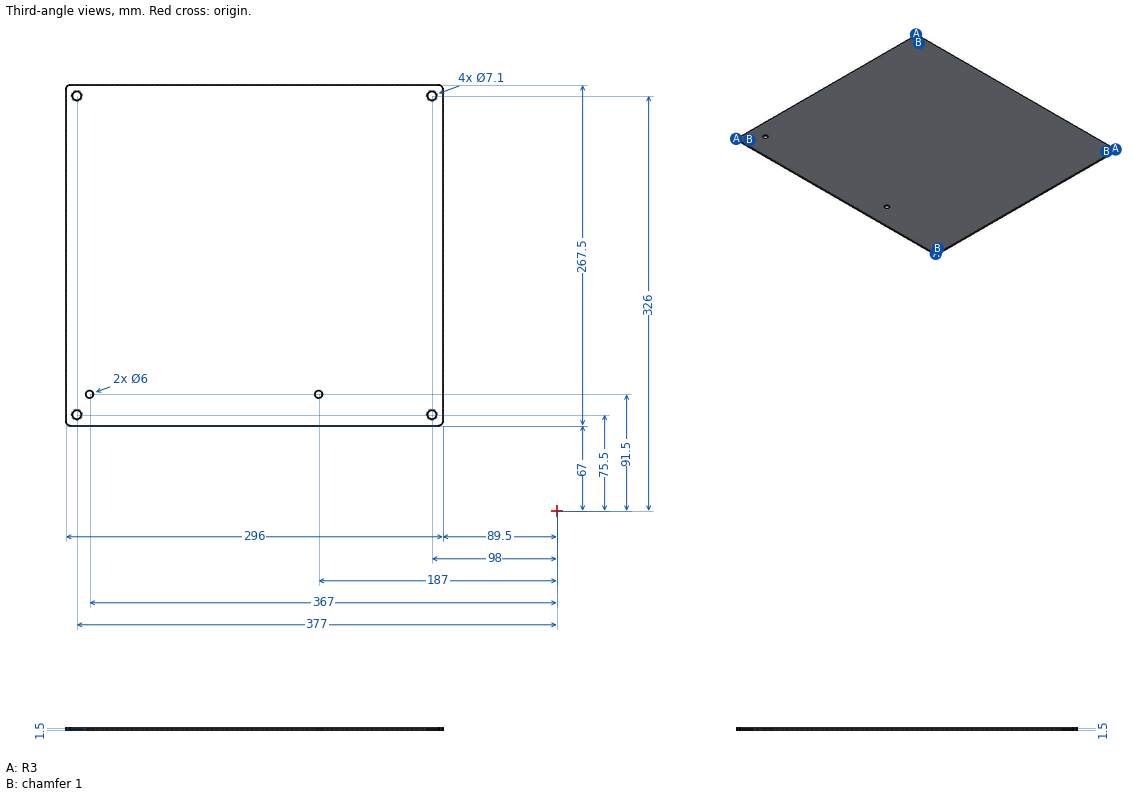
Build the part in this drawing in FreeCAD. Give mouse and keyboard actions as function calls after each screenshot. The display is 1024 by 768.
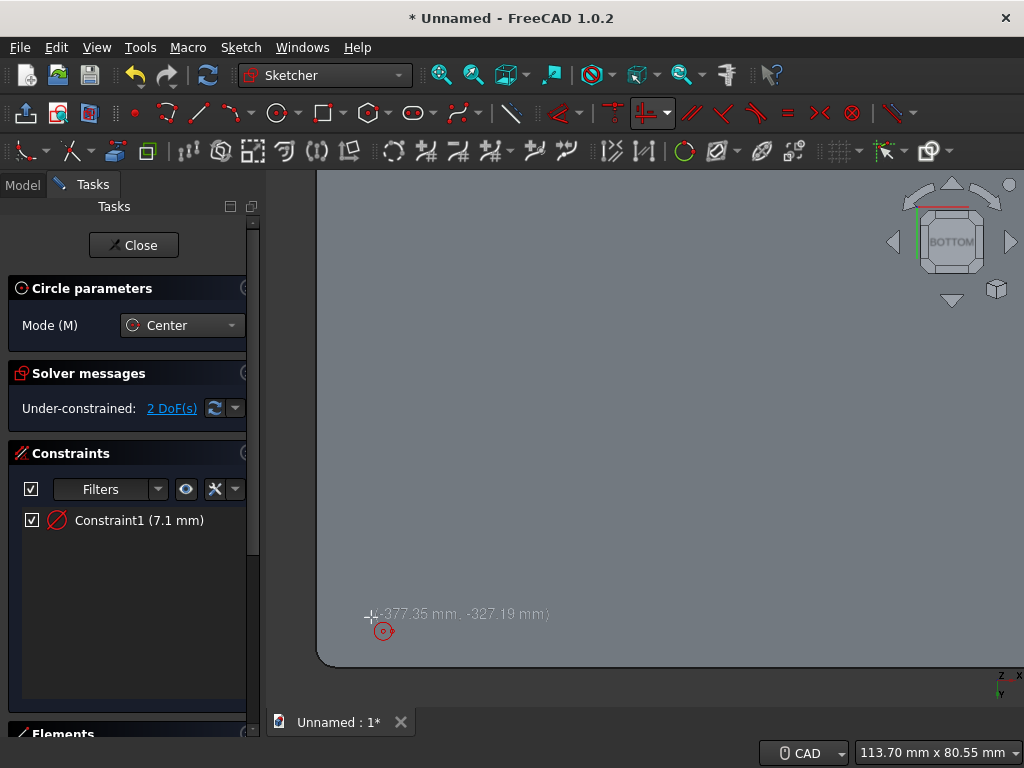
scroll(370, 617, down, 9)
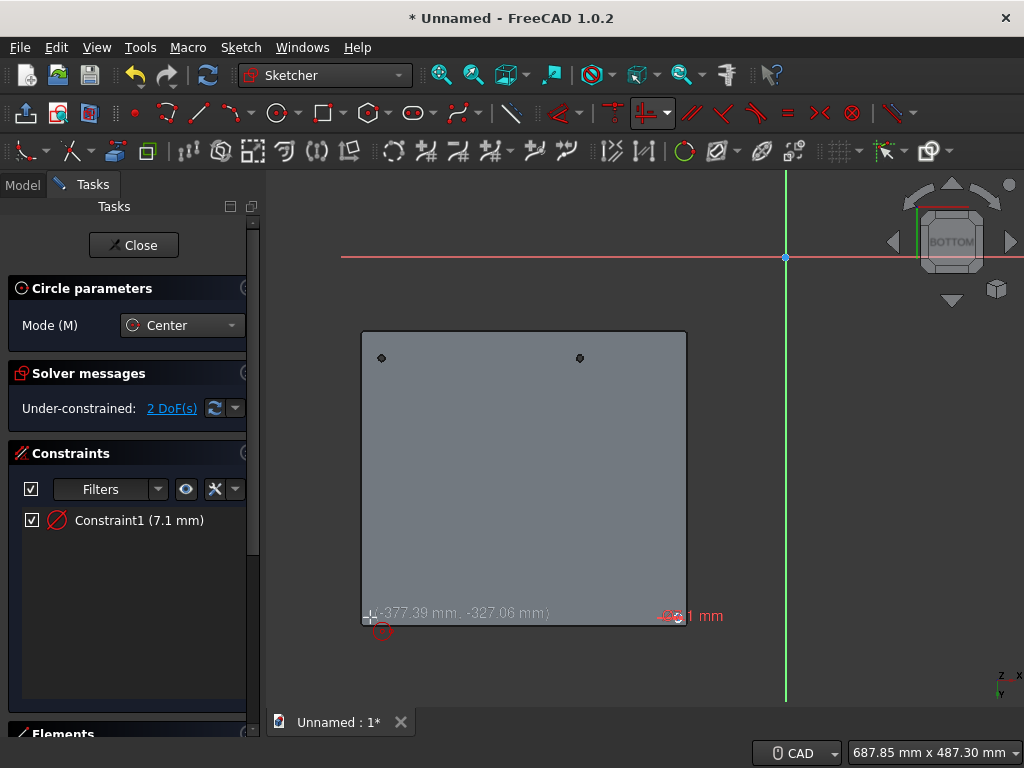
click(371, 617)
move(373, 614)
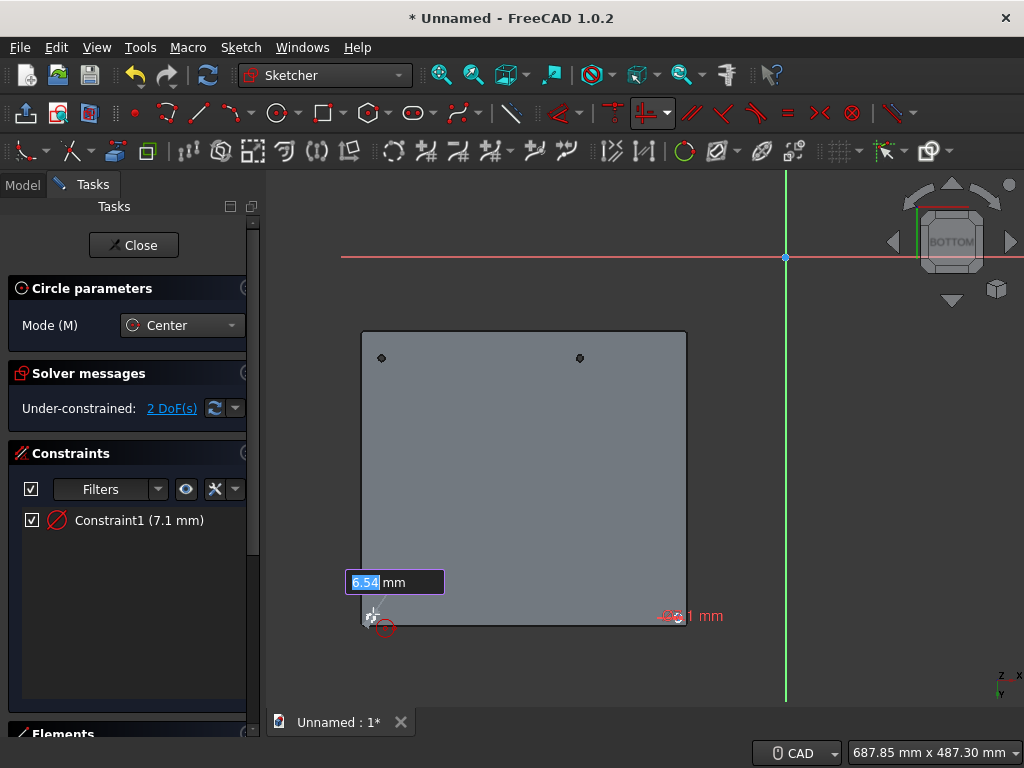
text(7.1)
key(Return)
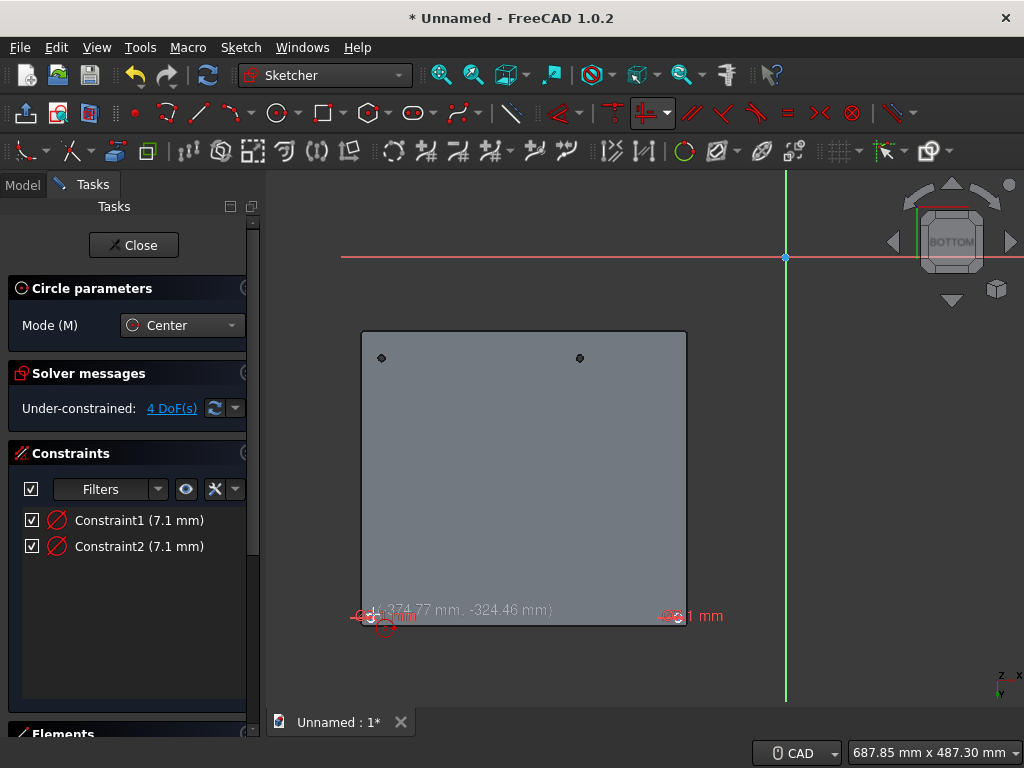
scroll(371, 341, up, 9)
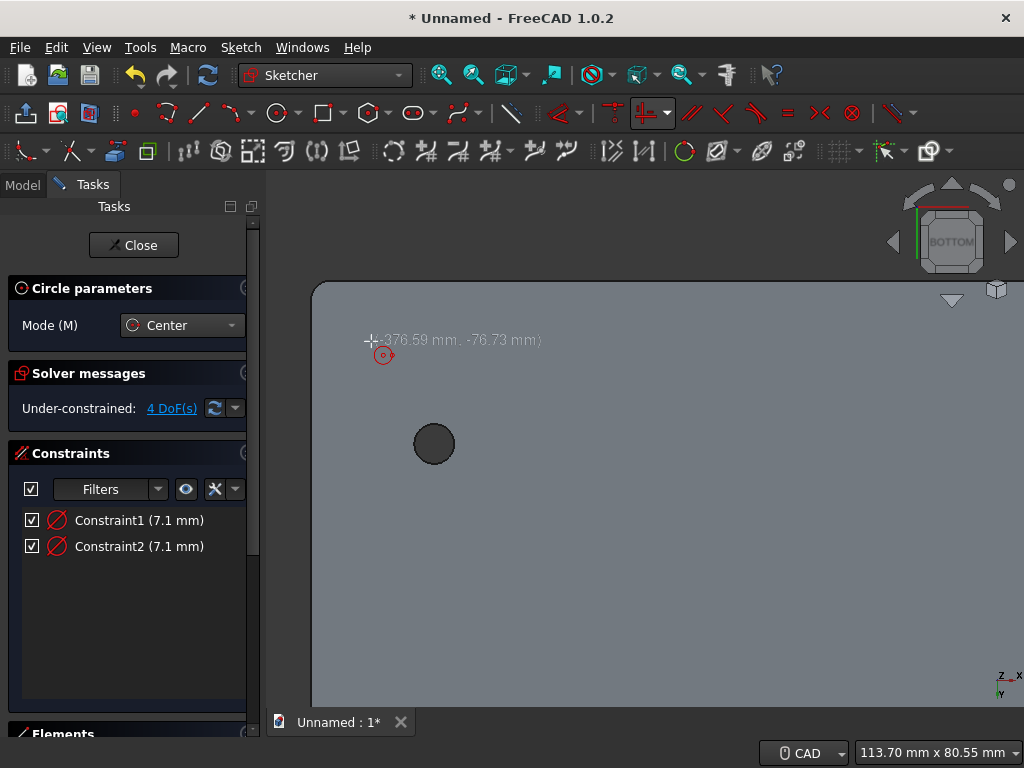
scroll(371, 341, down, 9)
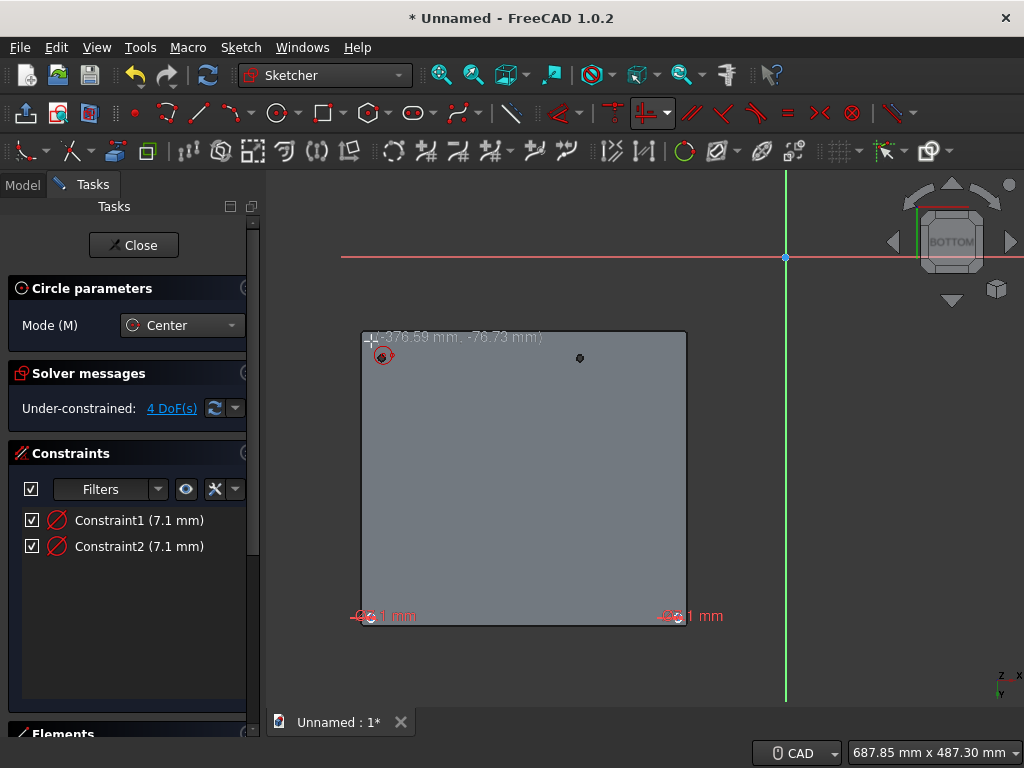
click(371, 341)
move(373, 338)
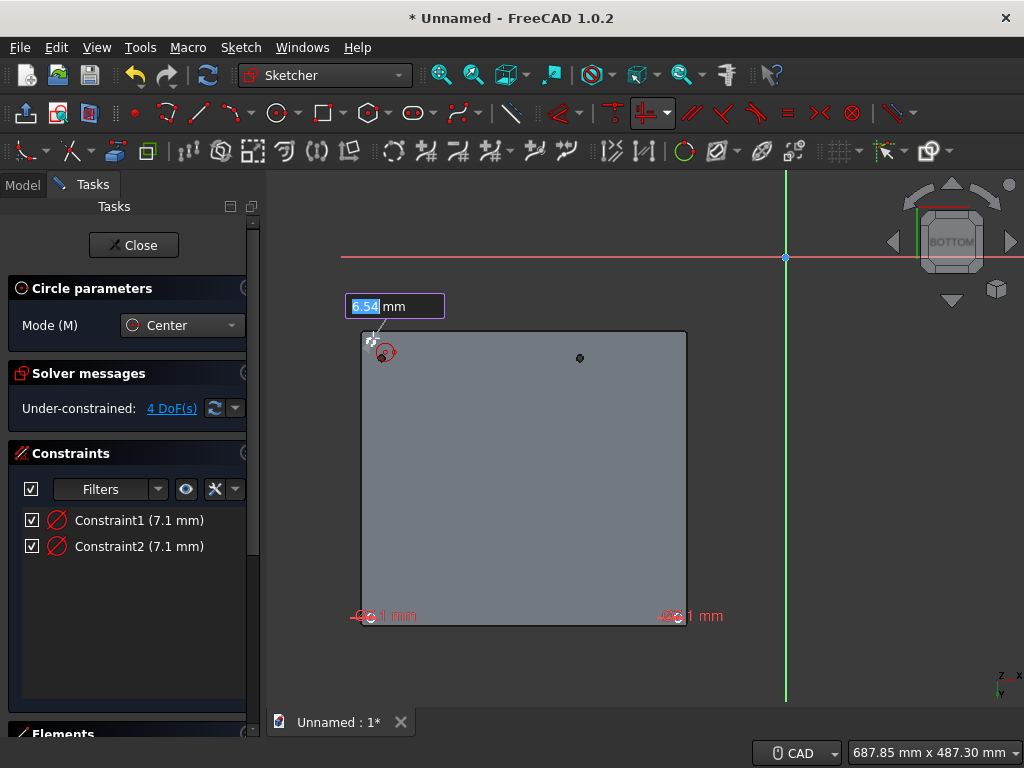
text(7.1)
key(Return)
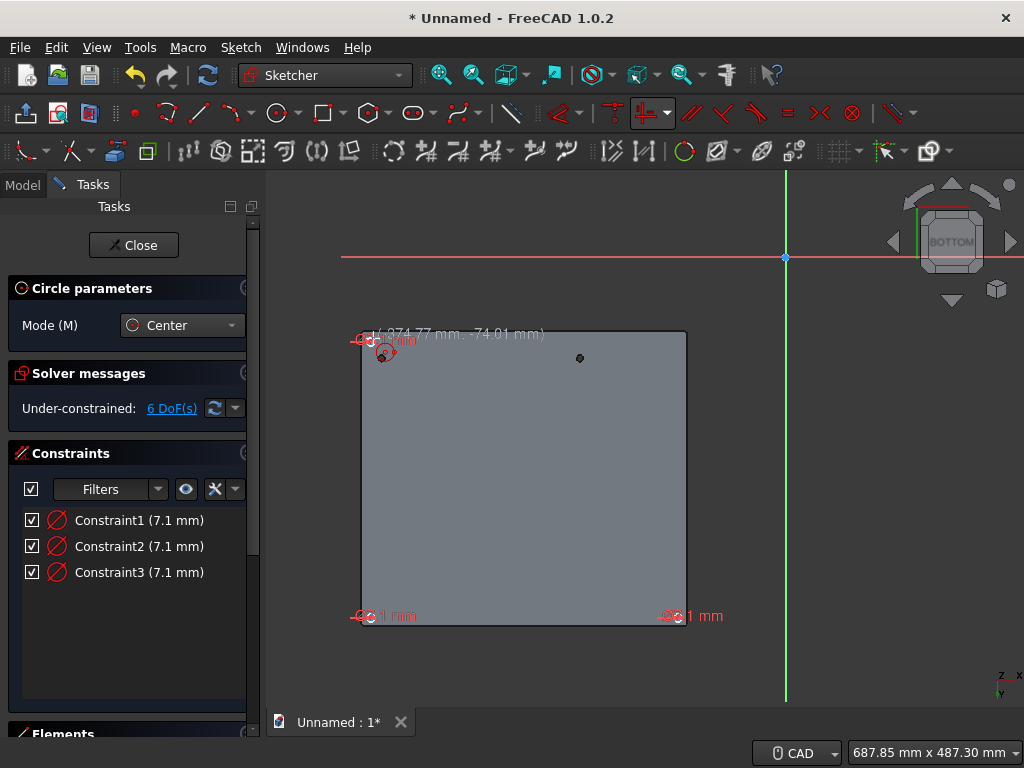
scroll(678, 341, up, 9)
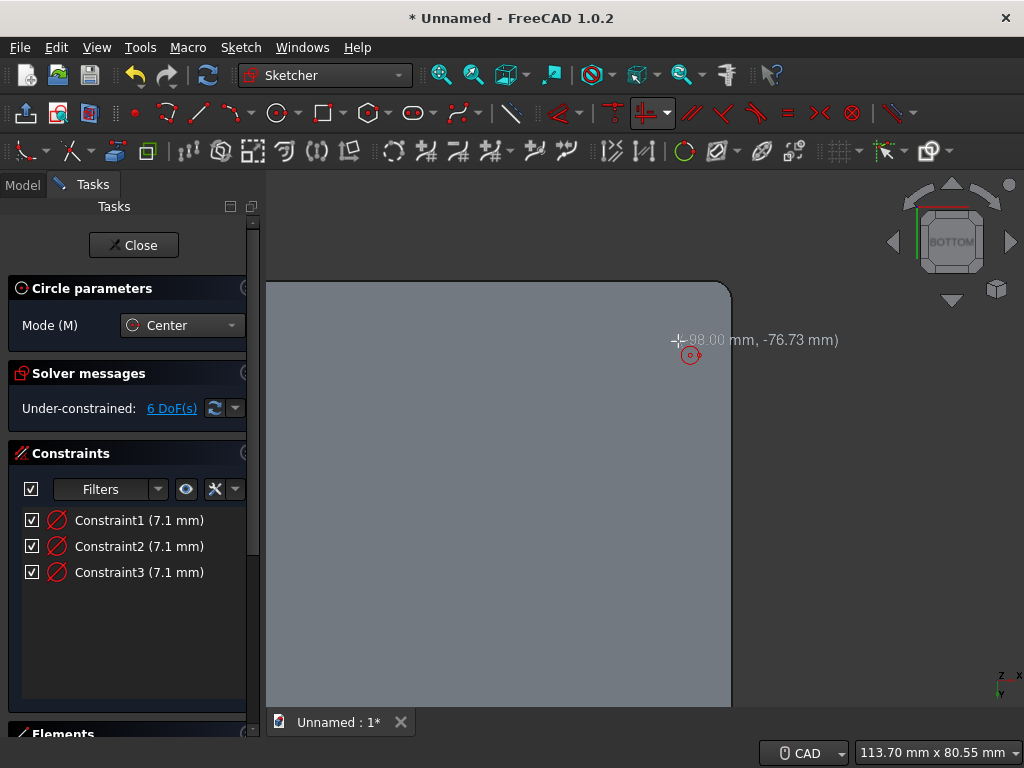
scroll(679, 341, down, 9)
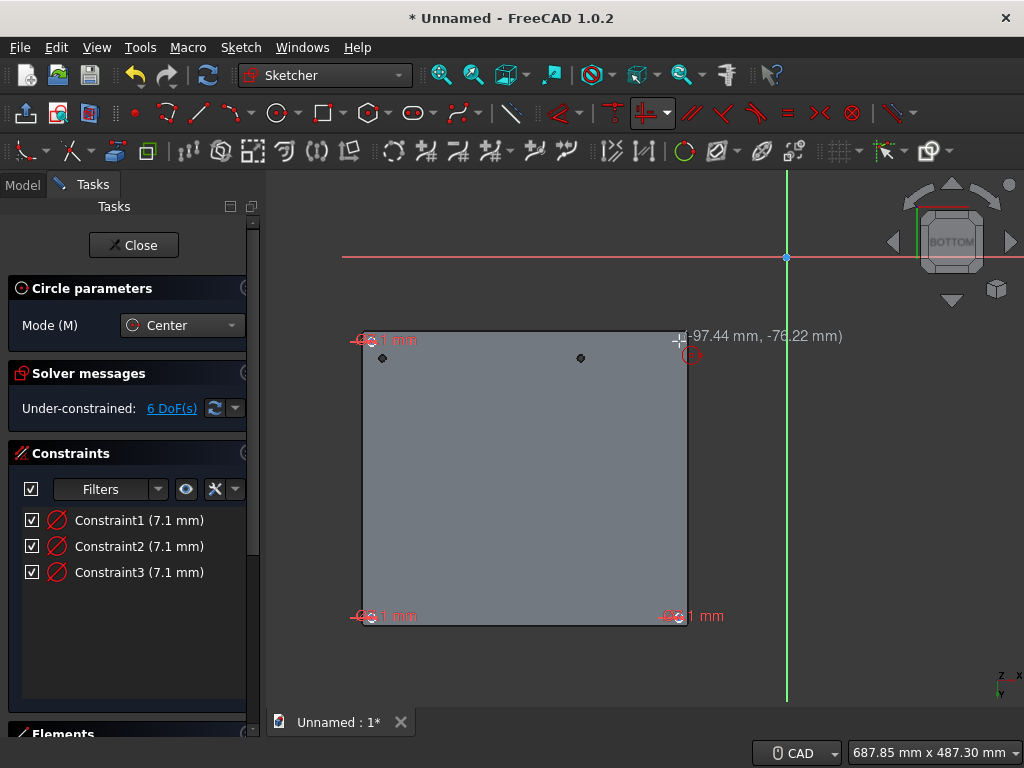
click(679, 341)
move(682, 338)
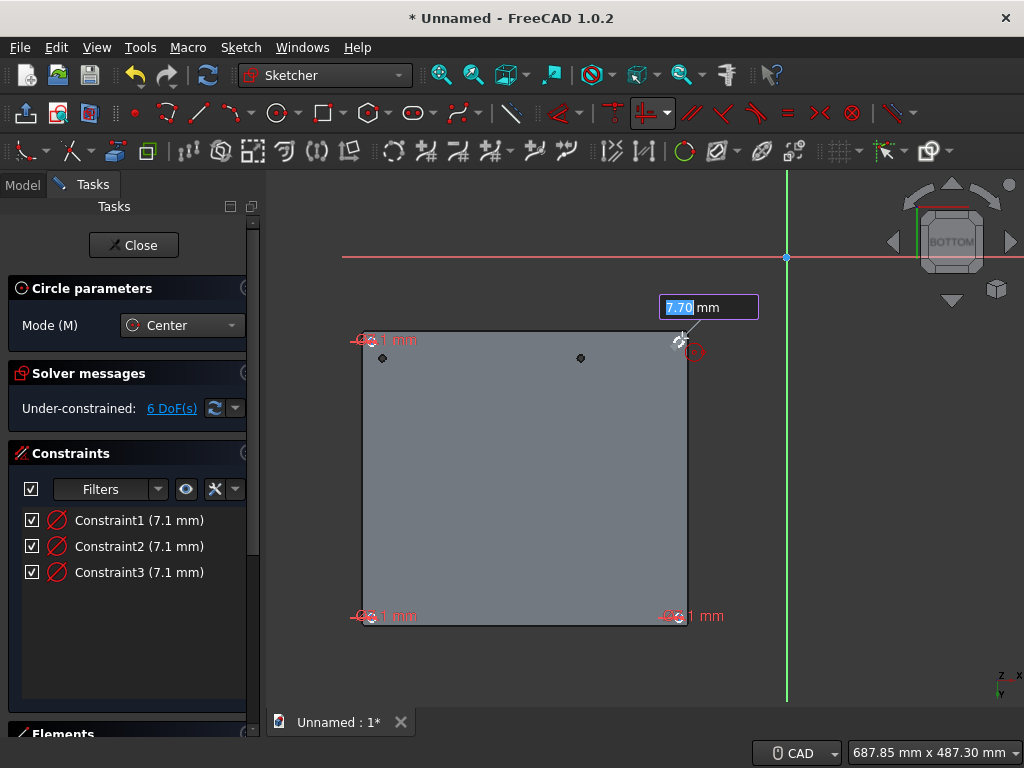
text(7.1)
key(Return)
key(Escape)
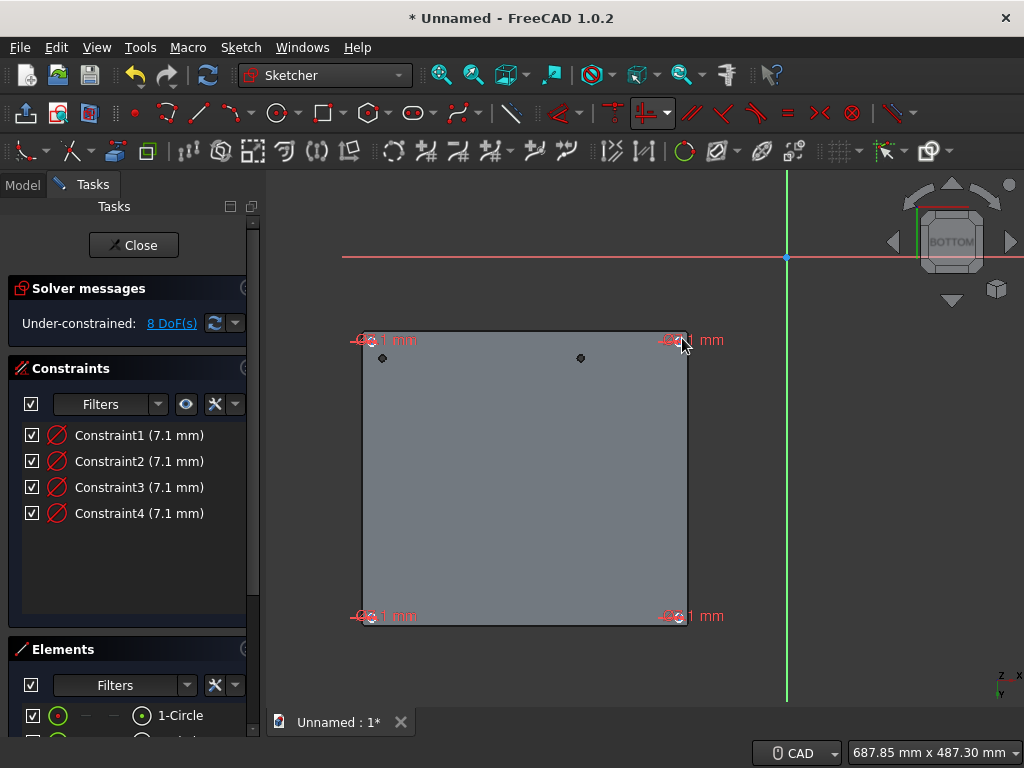
click(679, 618)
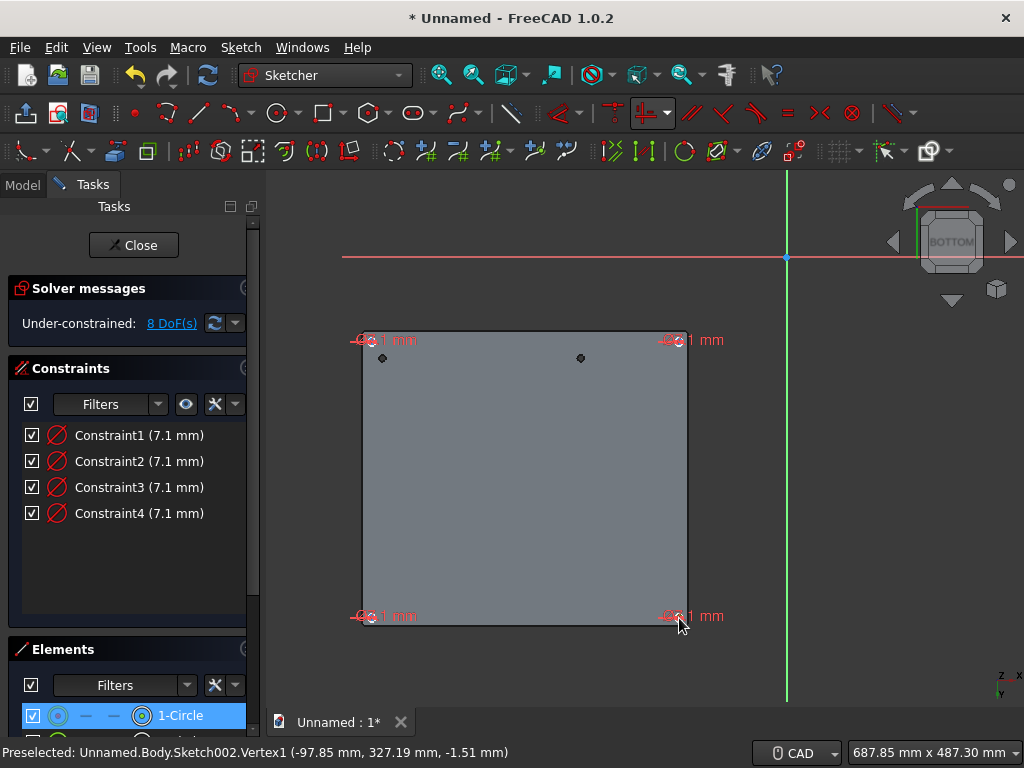
click(372, 618)